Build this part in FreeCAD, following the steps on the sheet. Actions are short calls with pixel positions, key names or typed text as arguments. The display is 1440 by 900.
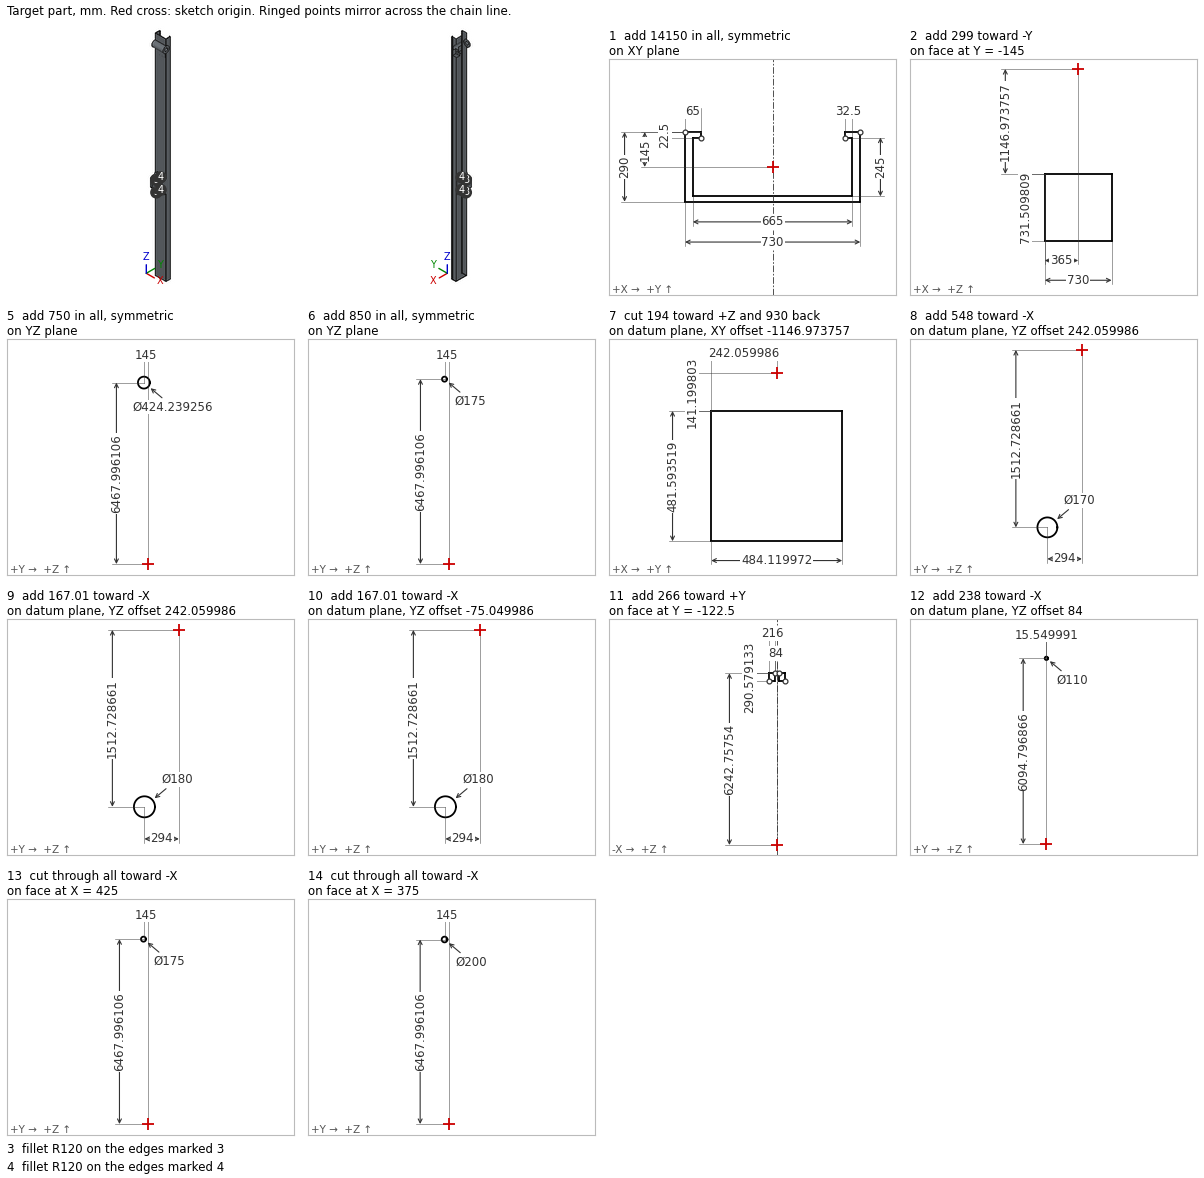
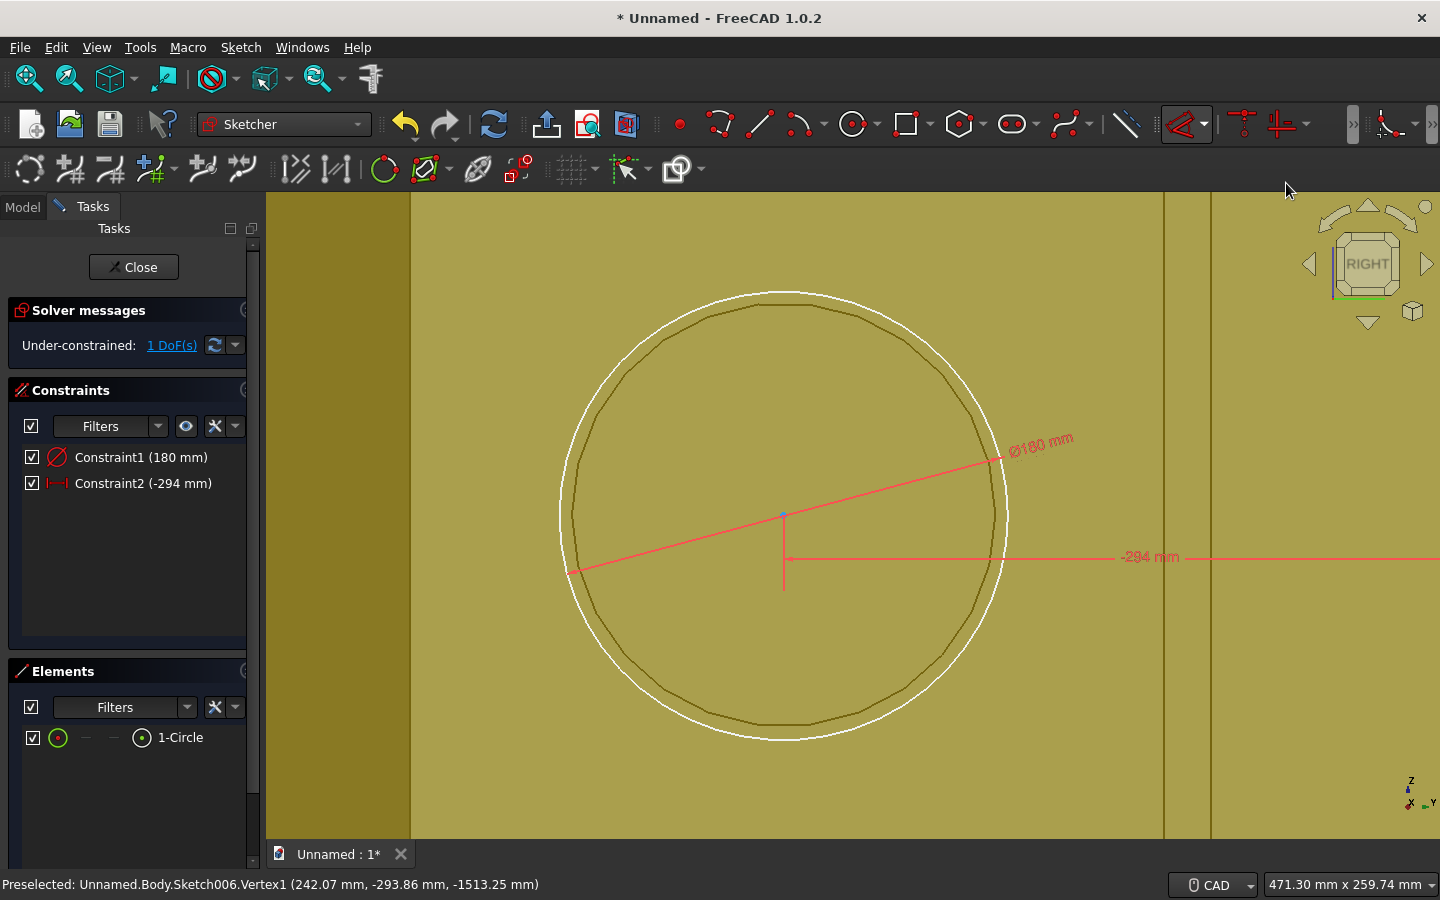
click(784, 516)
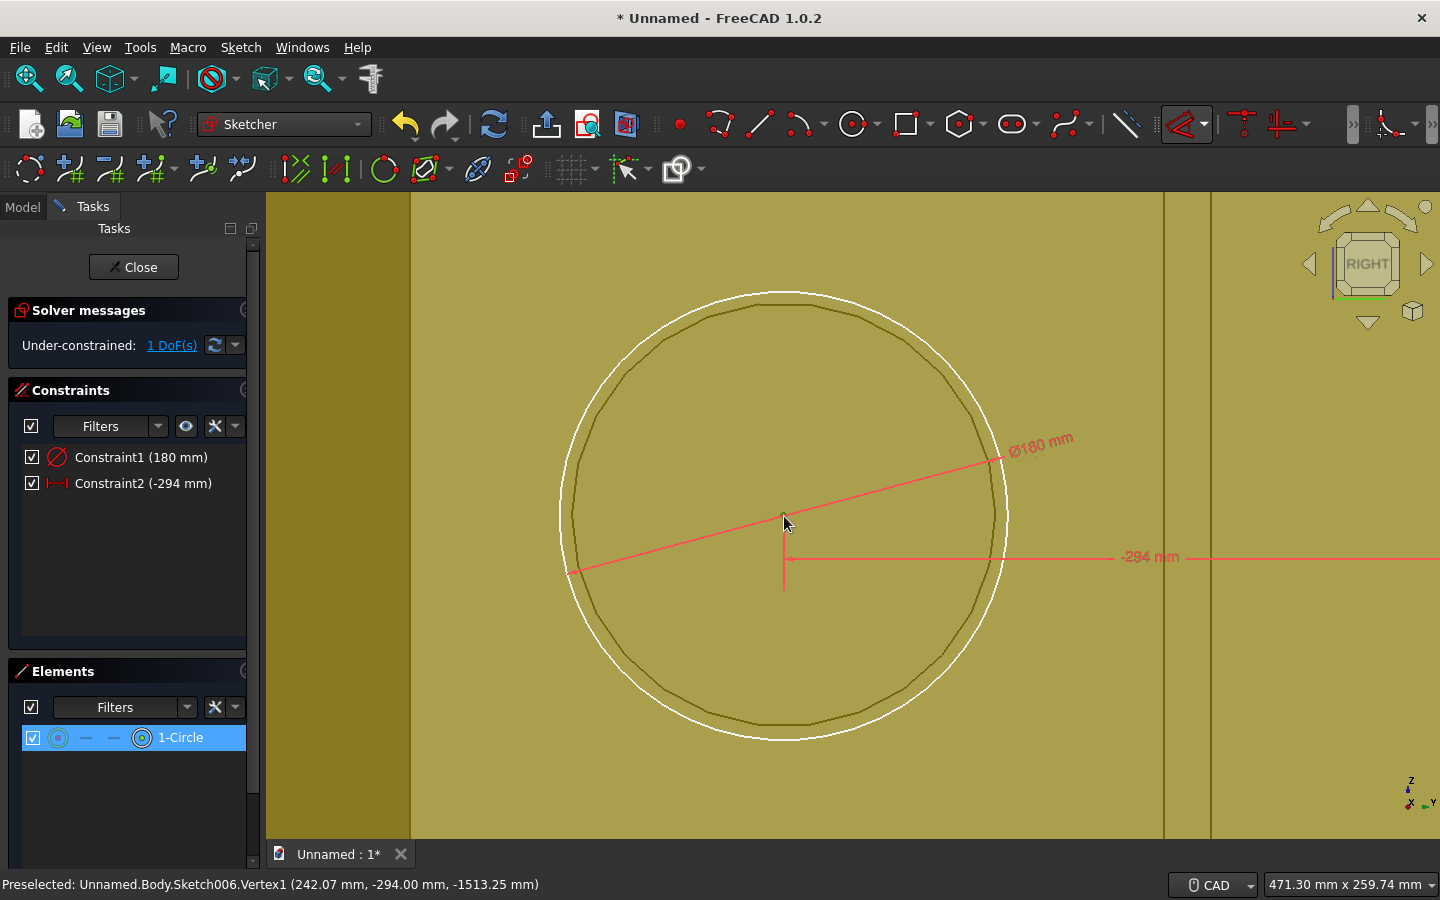
click(1206, 124)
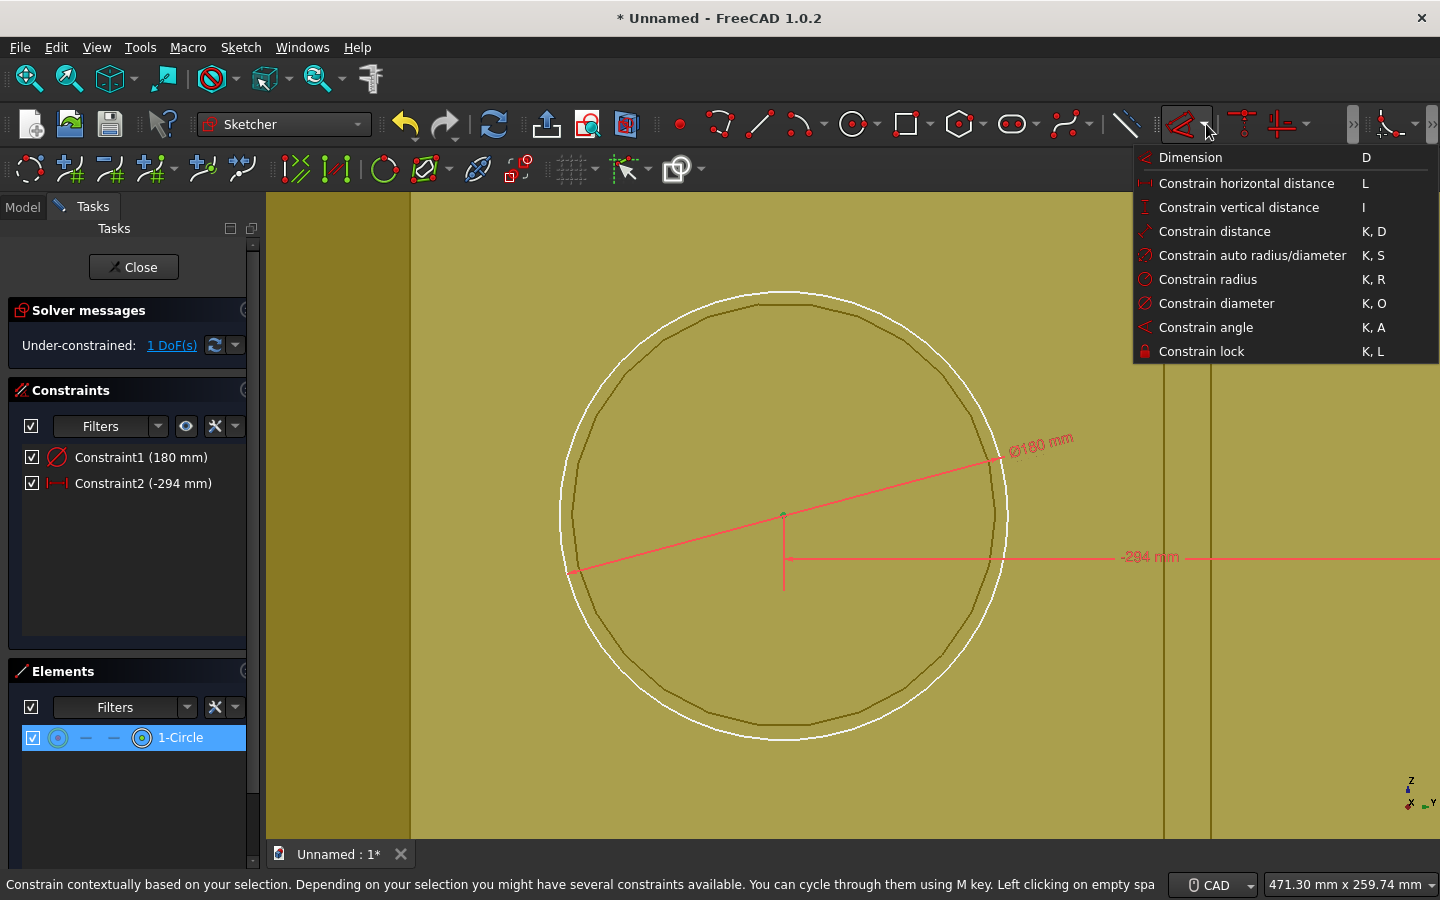
click(1286, 207)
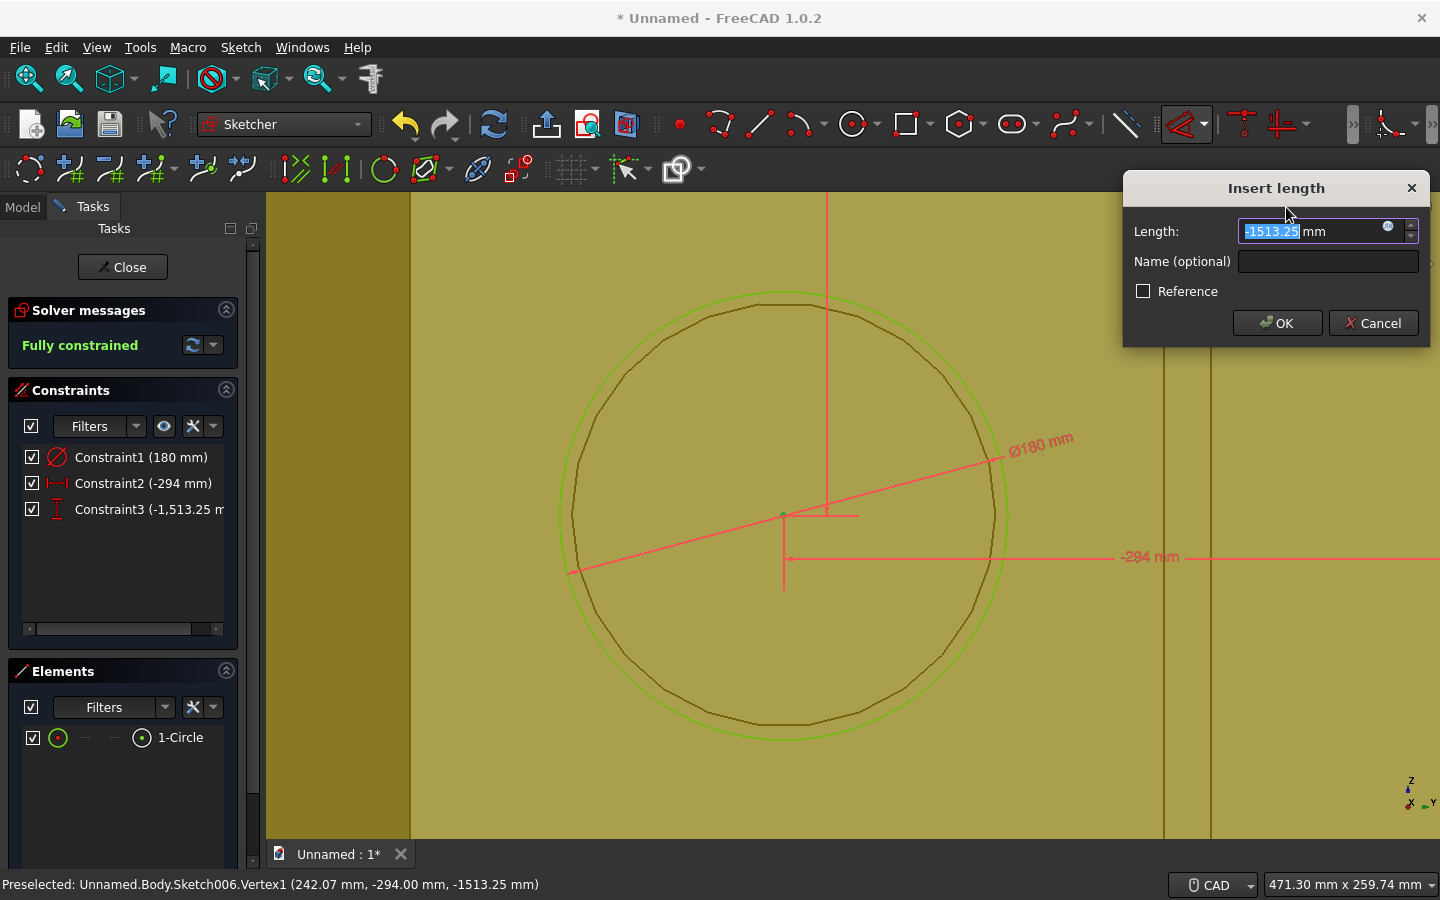
text(-1512.728661)
key(Return)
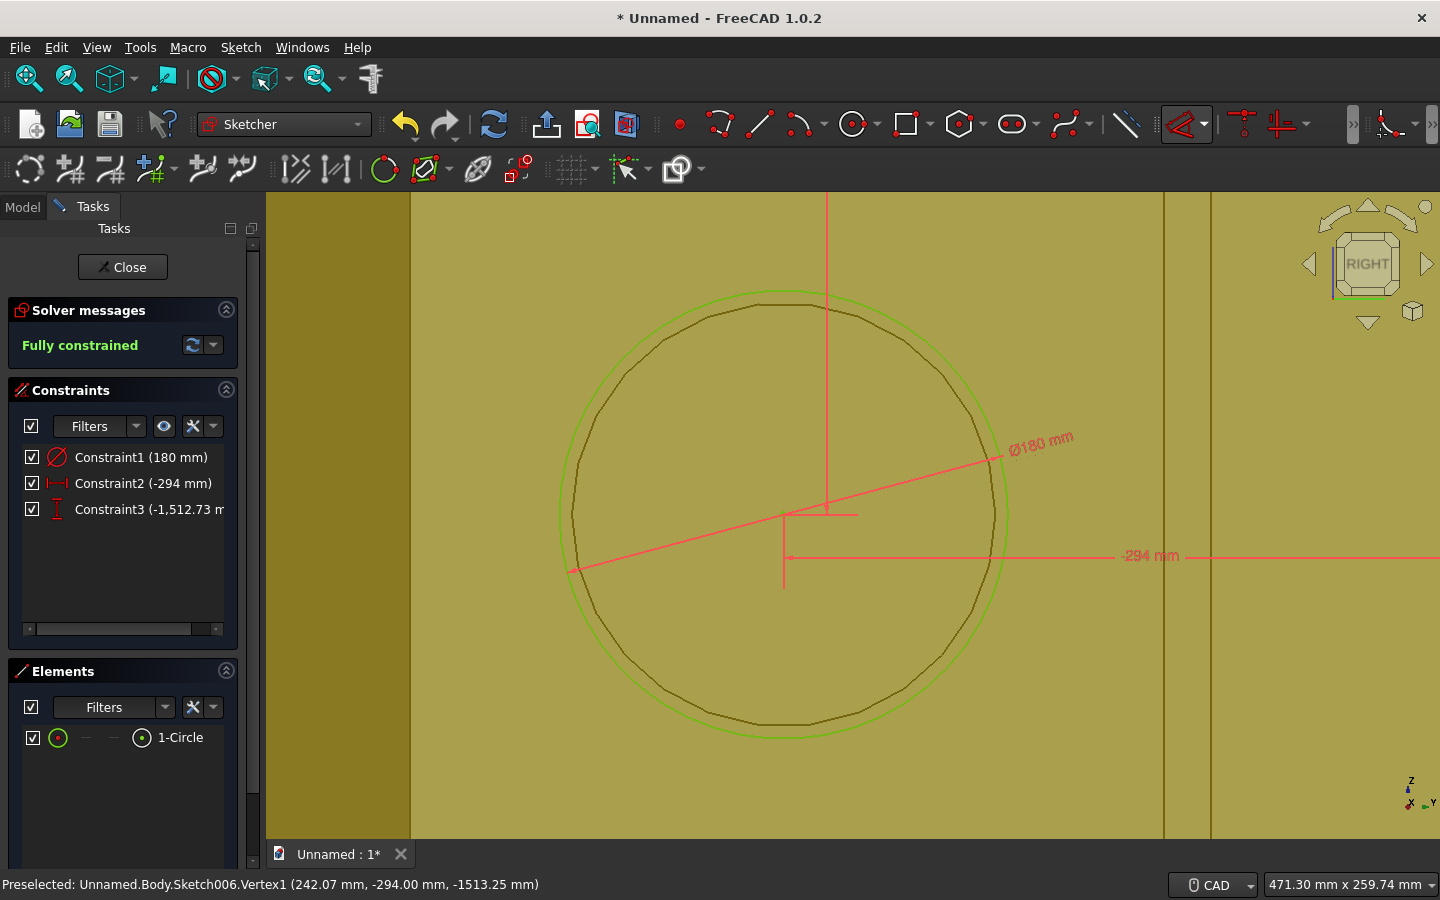
click(123, 267)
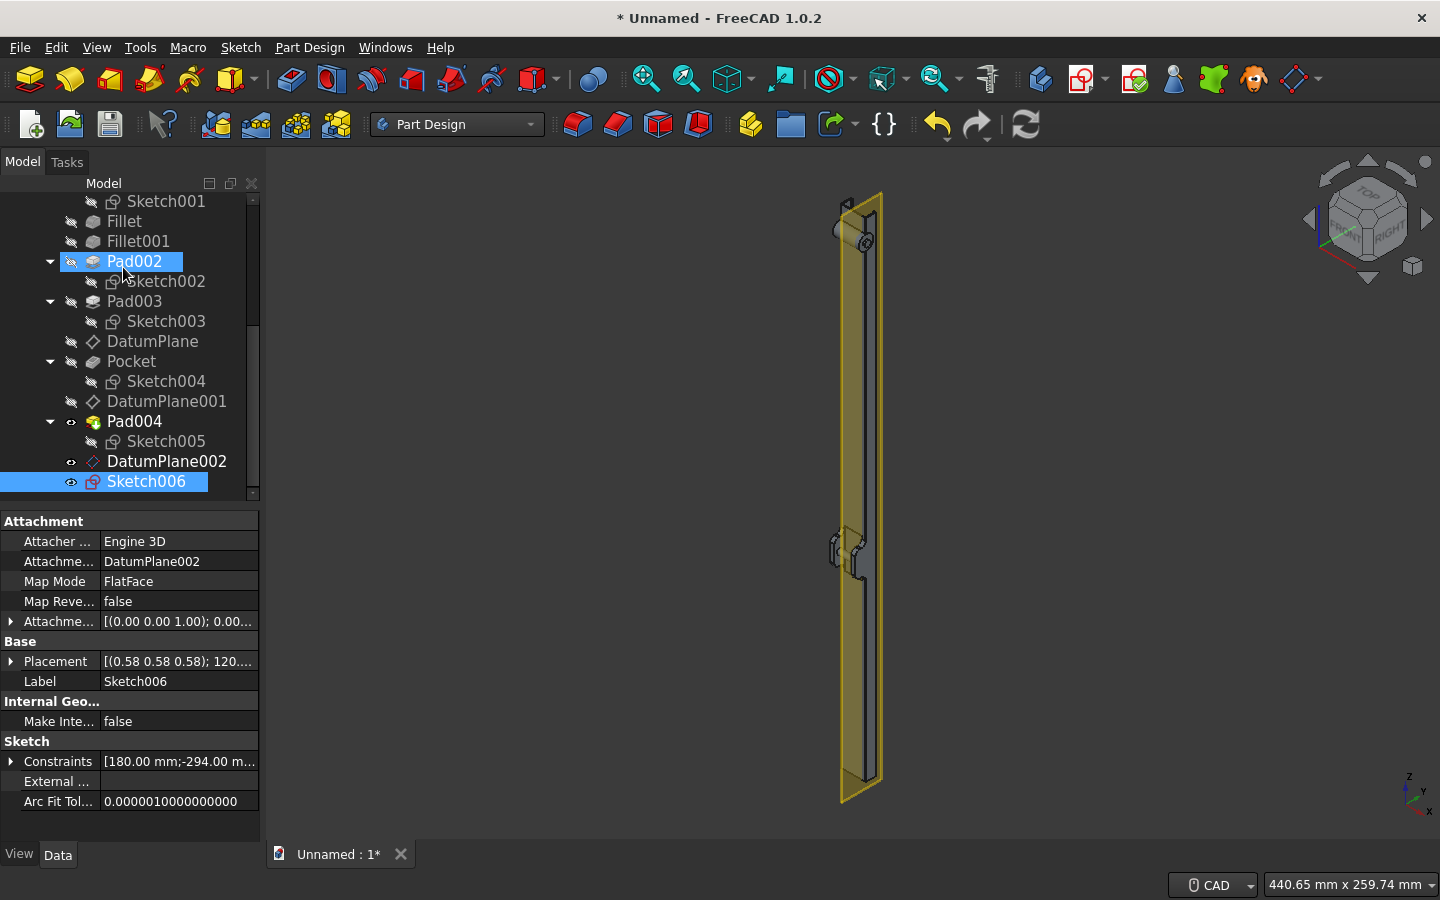
click(30, 80)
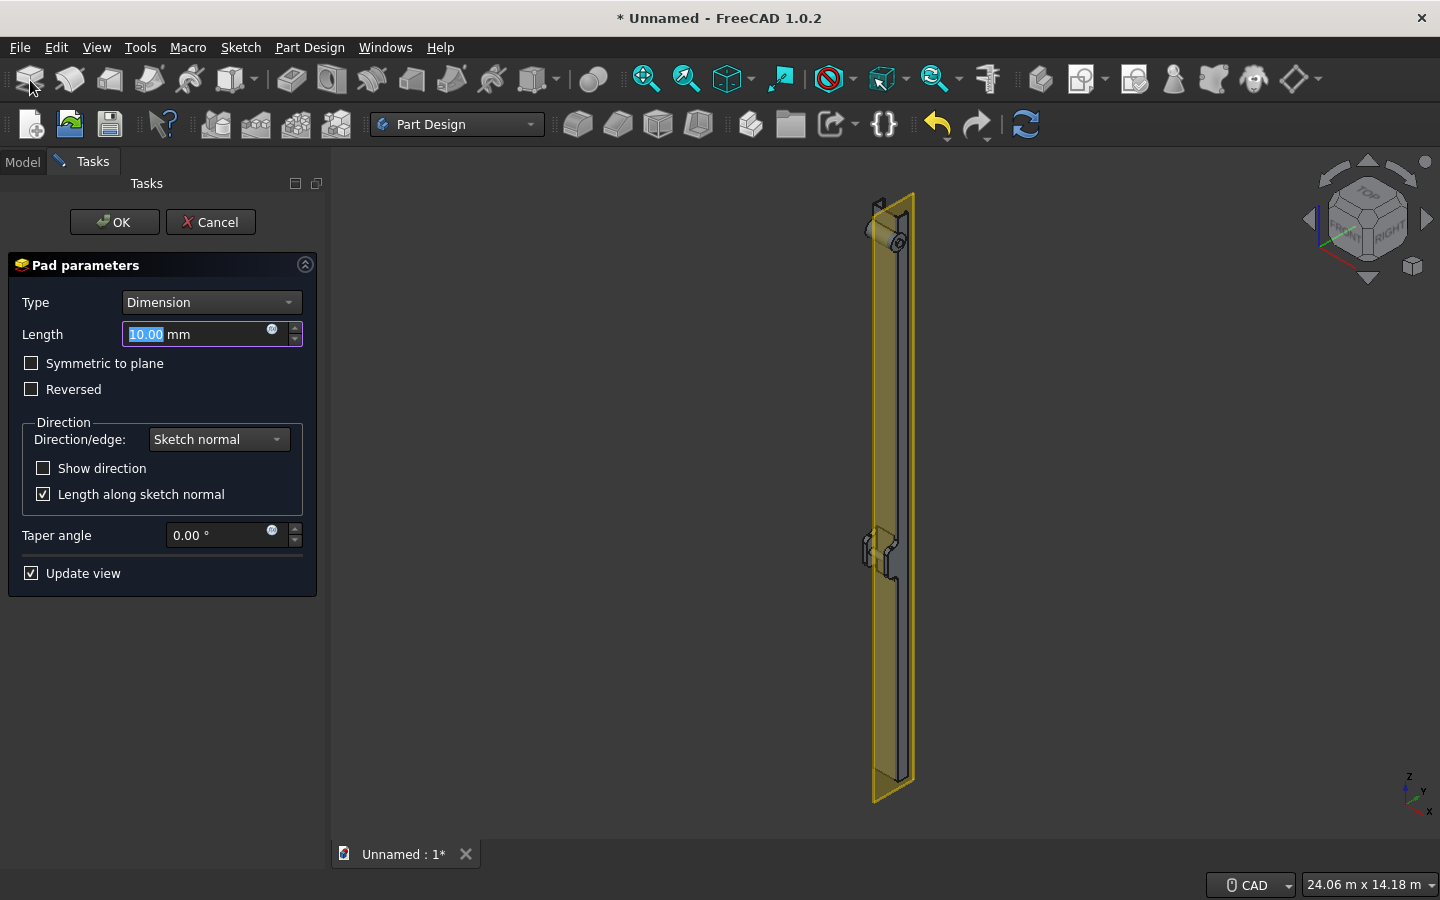
text(167.01)
key(Tab)